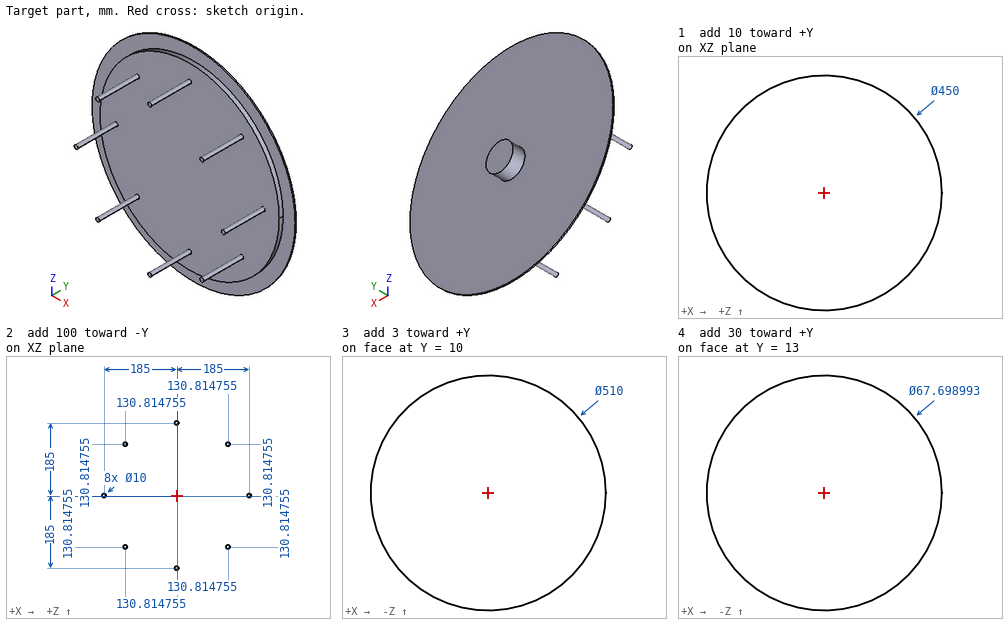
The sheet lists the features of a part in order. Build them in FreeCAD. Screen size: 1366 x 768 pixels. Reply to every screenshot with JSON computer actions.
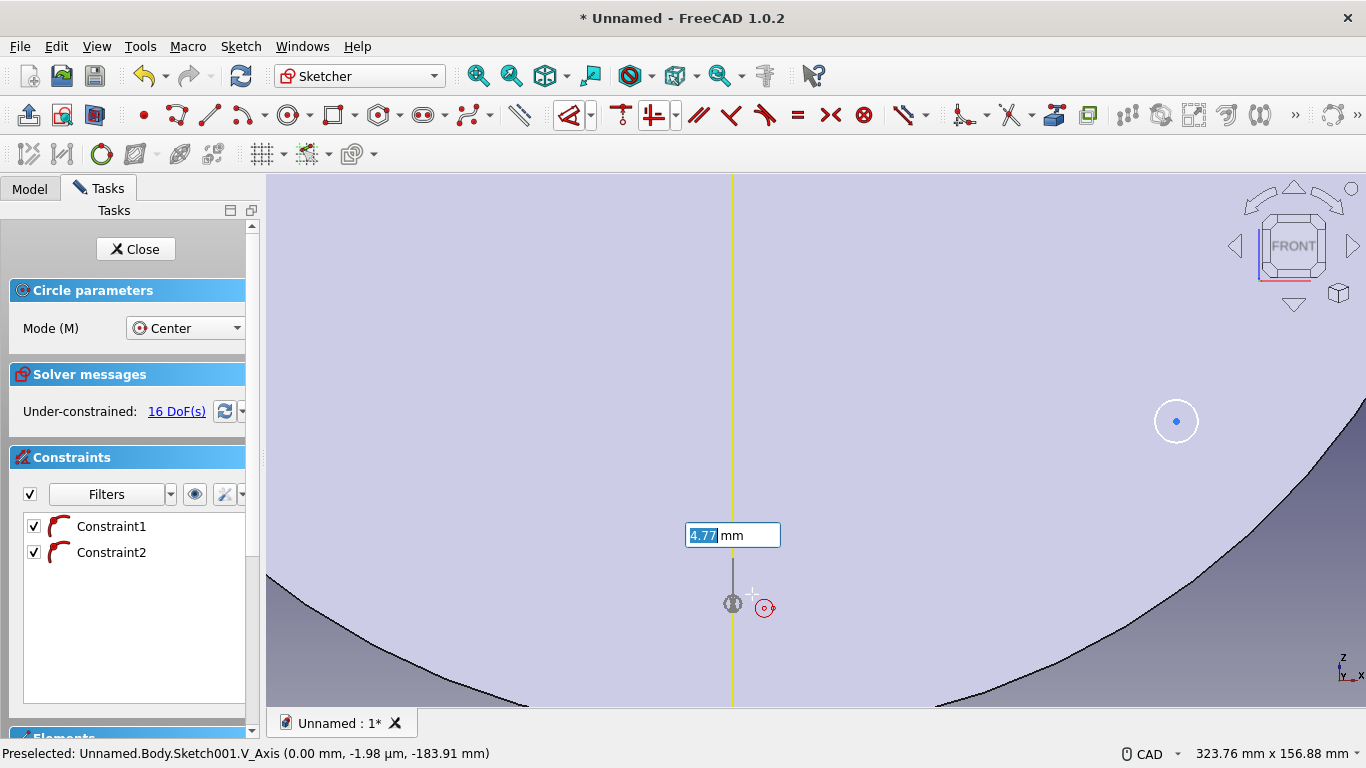
{"action": "left_click", "coordinate": [749, 594]}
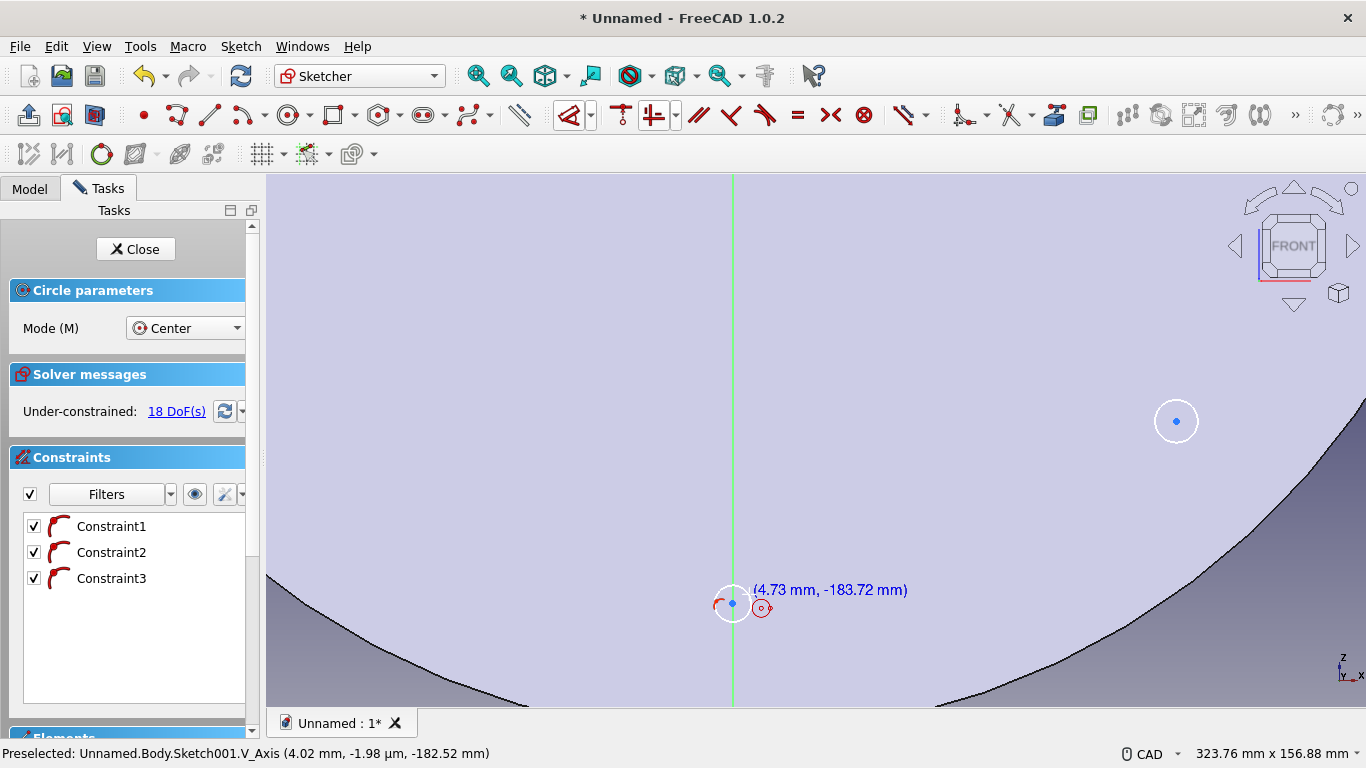
{"action": "scroll", "coordinate": [752, 594], "scroll_direction": "down", "scroll_amount": 7}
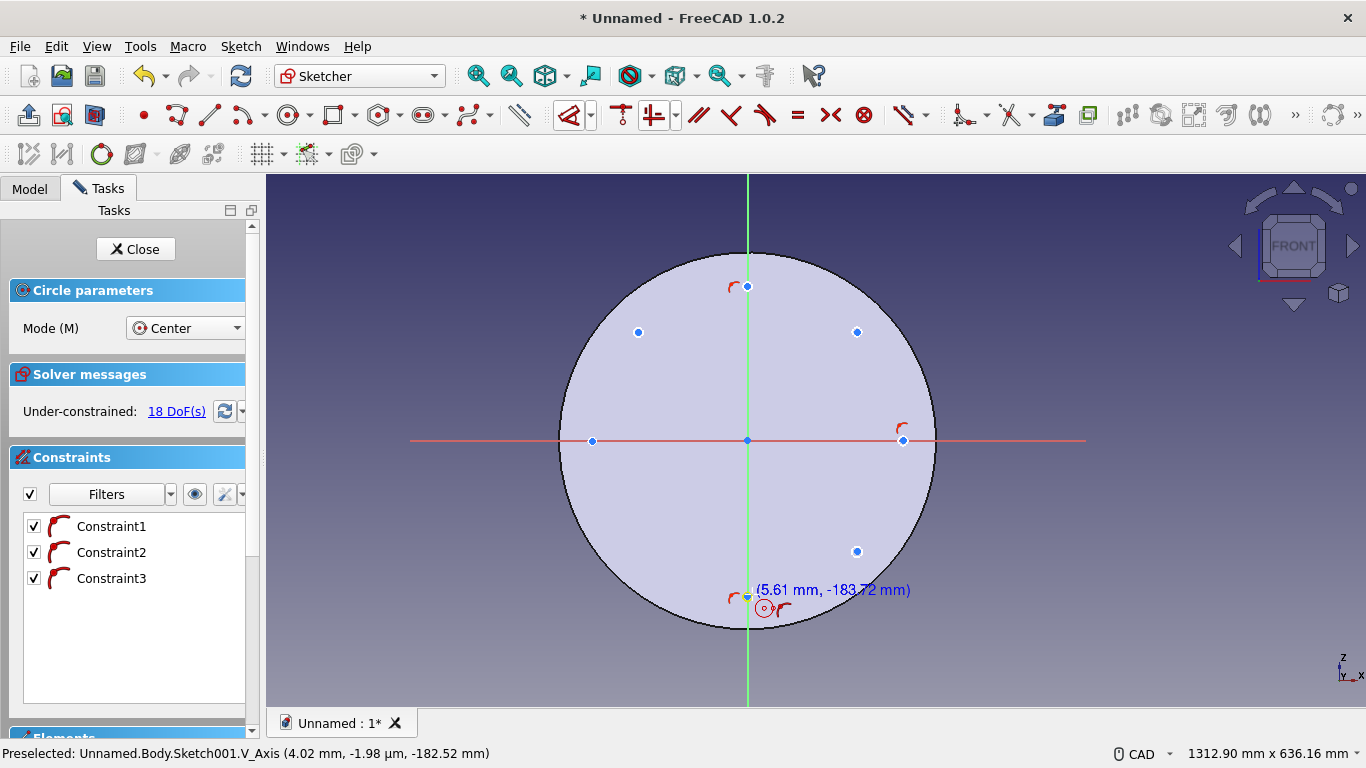
{"action": "scroll", "coordinate": [638, 551], "scroll_direction": "up", "scroll_amount": 9}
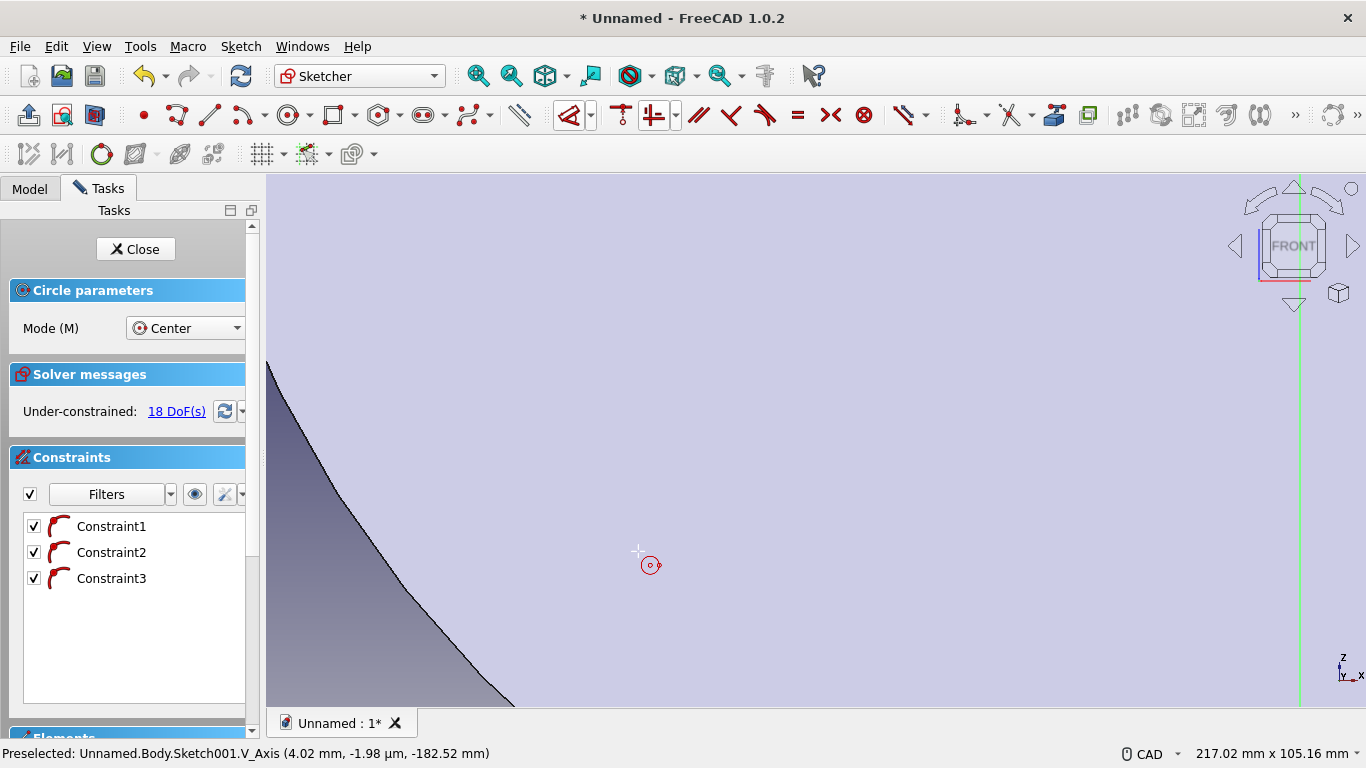
{"action": "scroll", "coordinate": [638, 551], "scroll_direction": "down", "scroll_amount": 9}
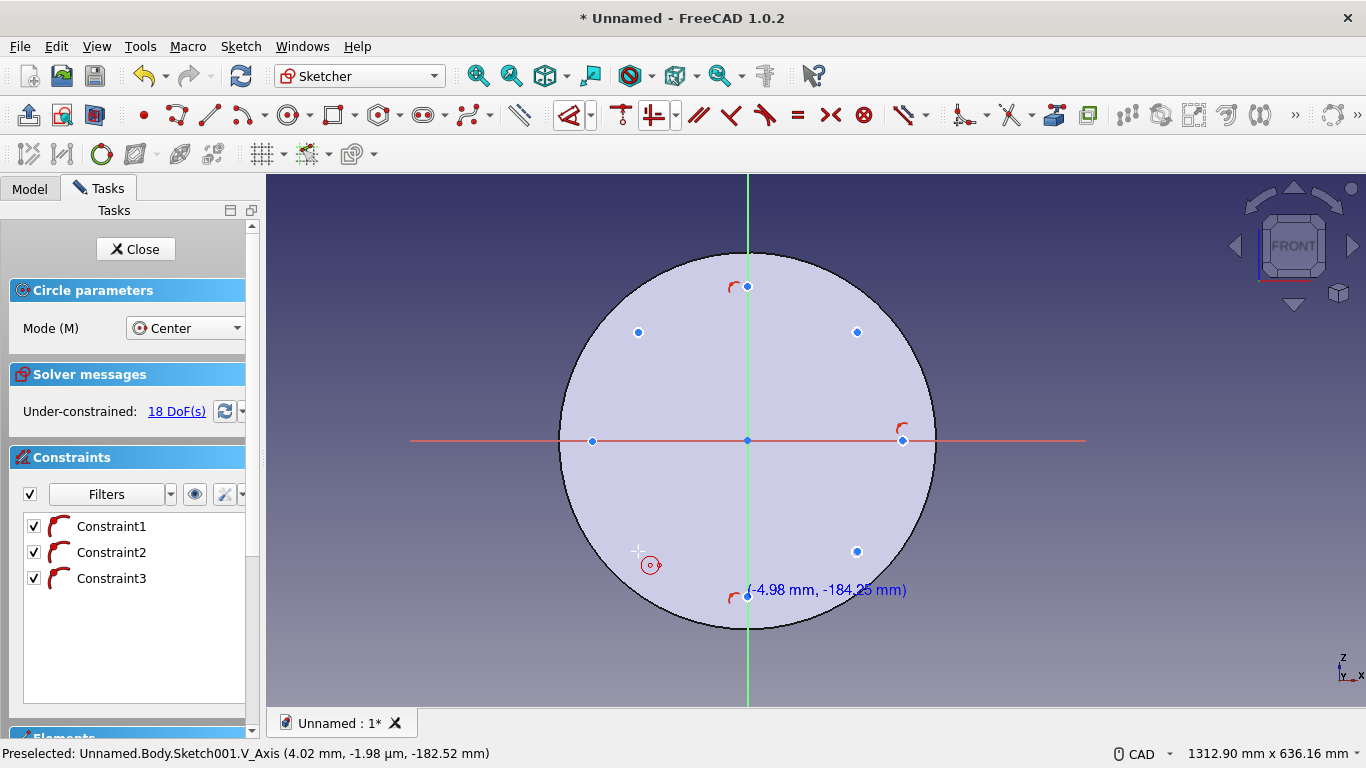
{"action": "left_click", "coordinate": [638, 551]}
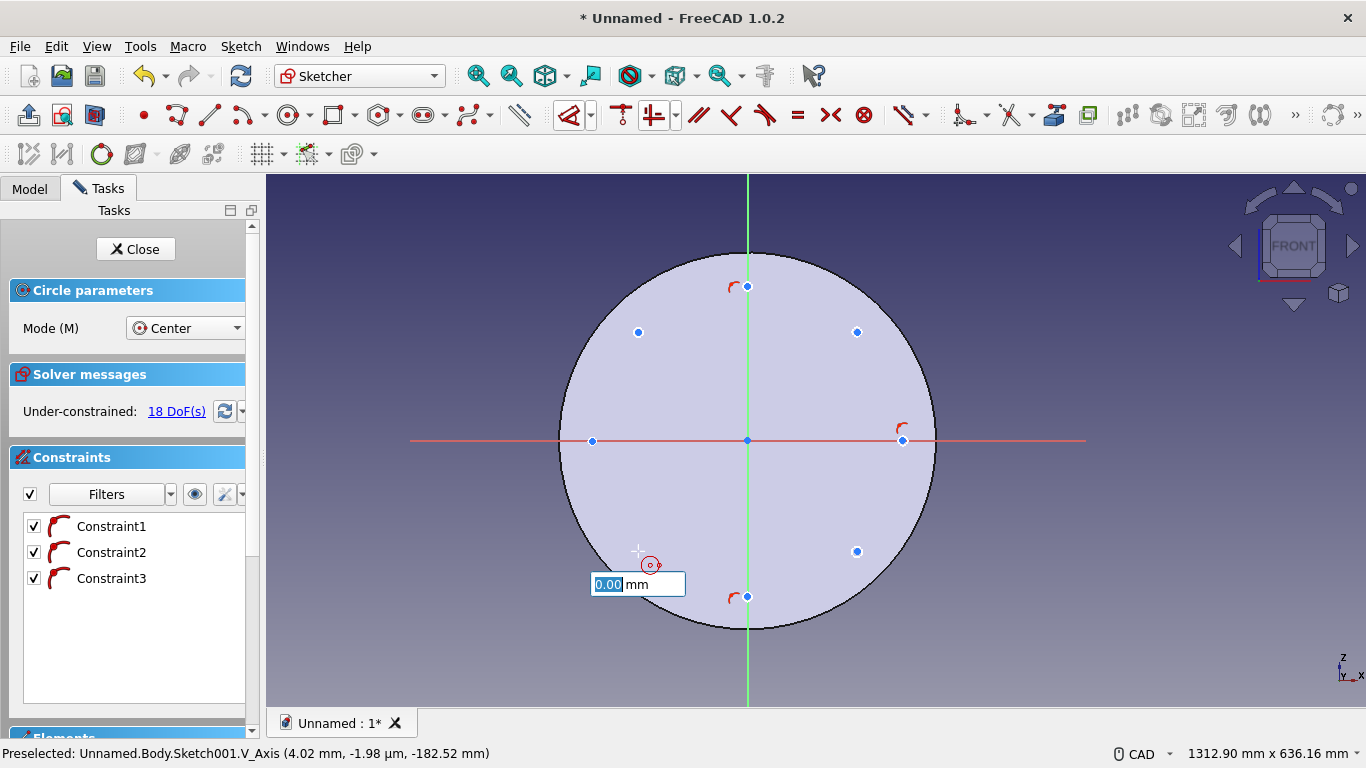
{"action": "scroll", "coordinate": [641, 548], "scroll_direction": "up", "scroll_amount": 7}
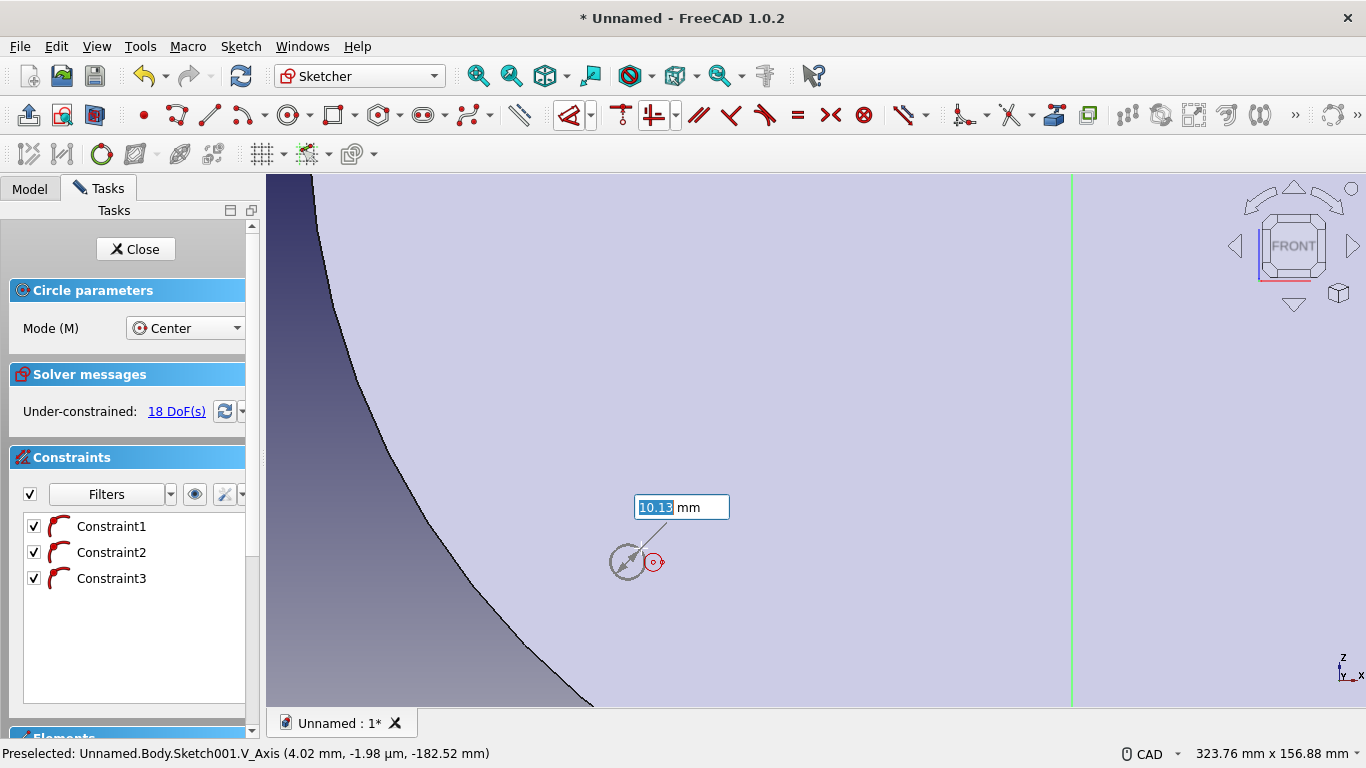
{"action": "left_click", "coordinate": [640, 544]}
{"action": "key", "text": "Escape"}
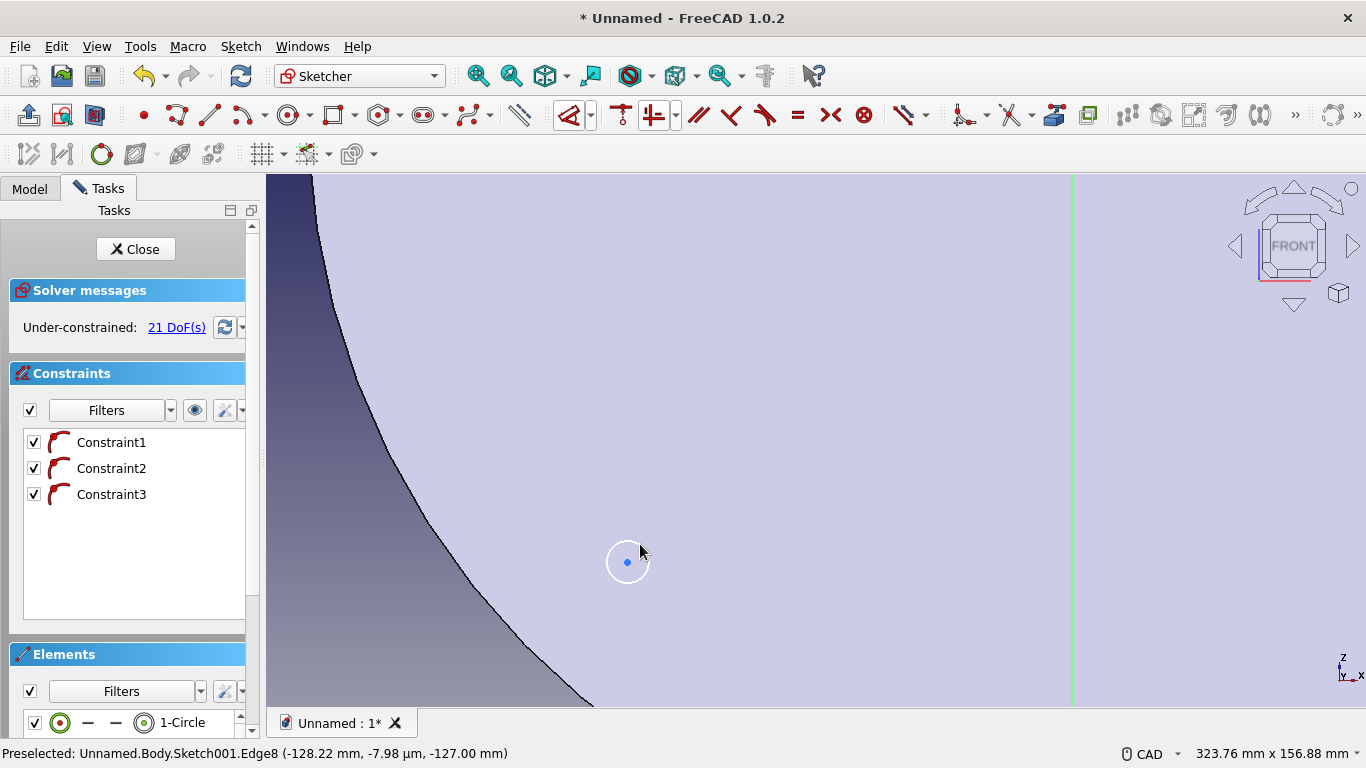
{"action": "scroll", "coordinate": [641, 548], "scroll_direction": "down", "scroll_amount": 7}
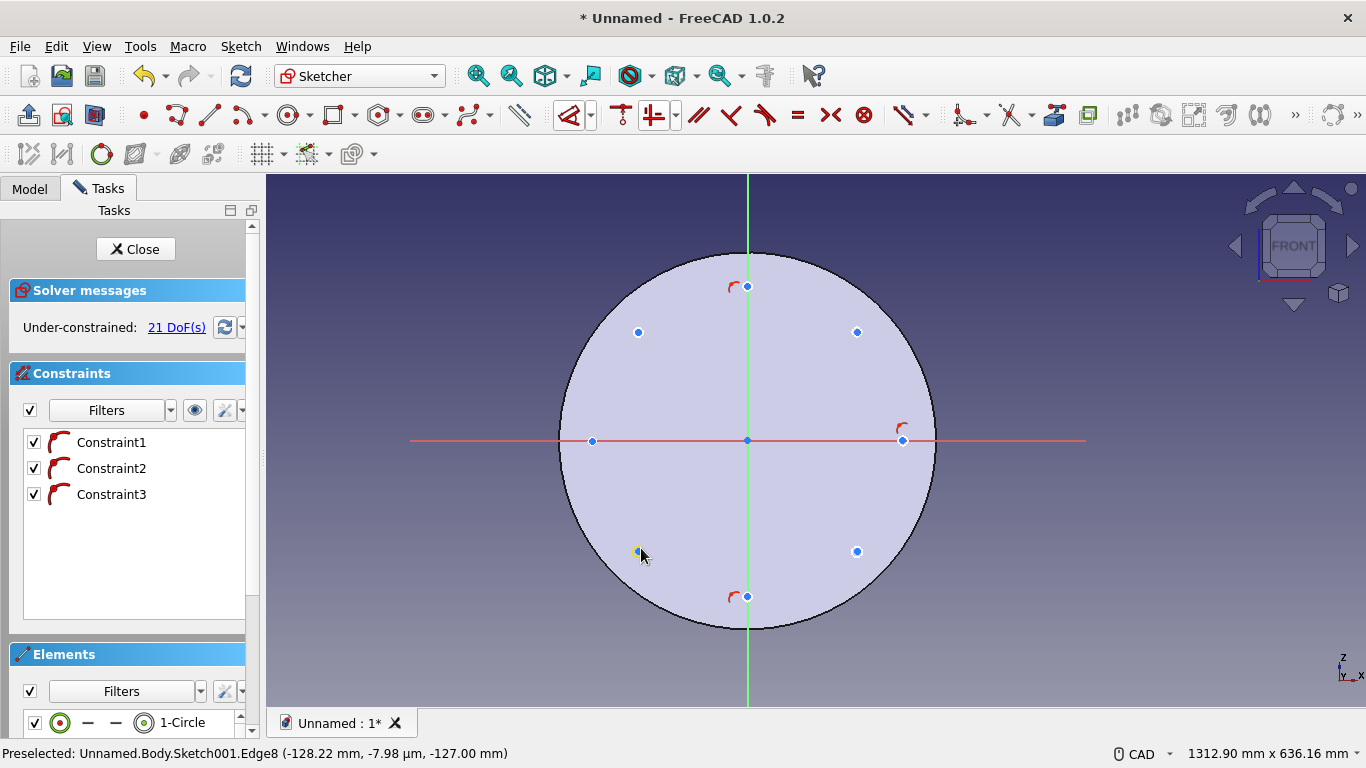
{"action": "scroll", "coordinate": [590, 444], "scroll_direction": "up", "scroll_amount": 8}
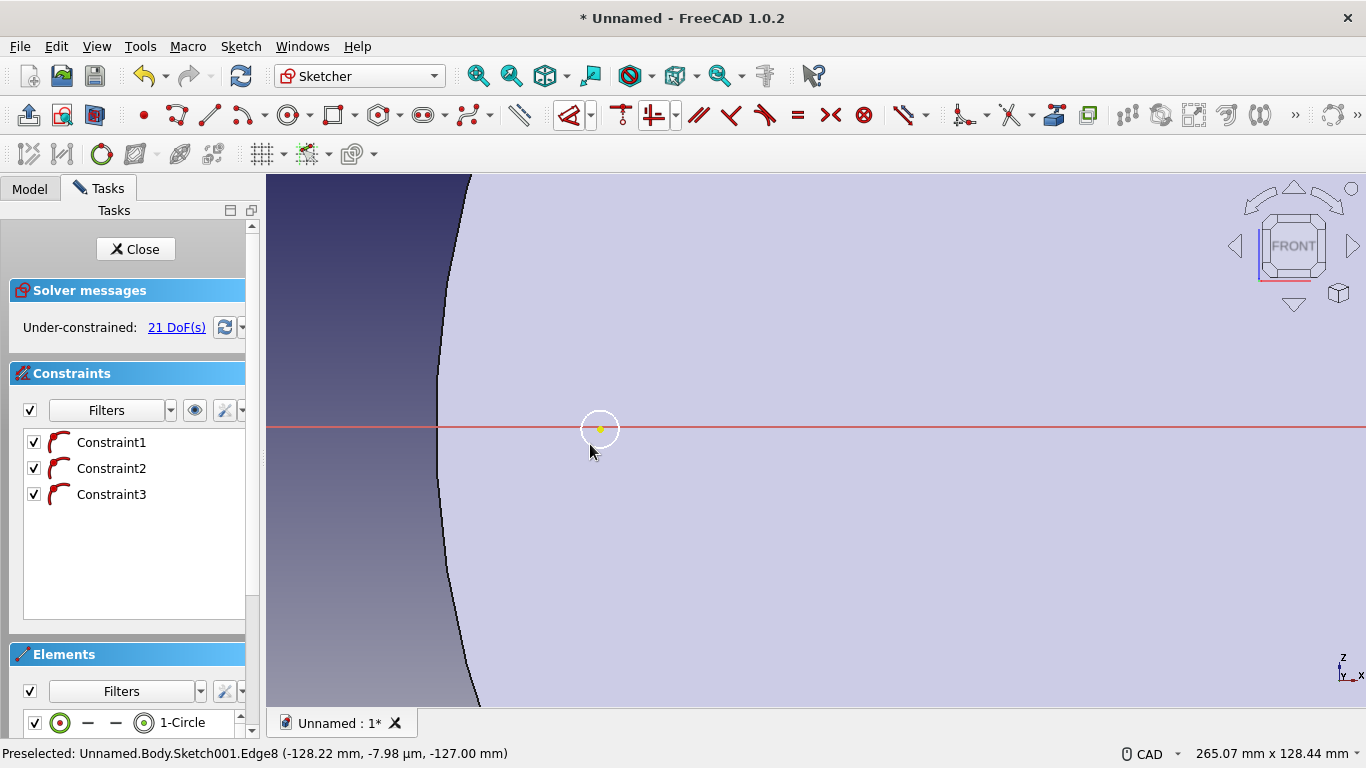
{"action": "left_click", "coordinate": [587, 442]}